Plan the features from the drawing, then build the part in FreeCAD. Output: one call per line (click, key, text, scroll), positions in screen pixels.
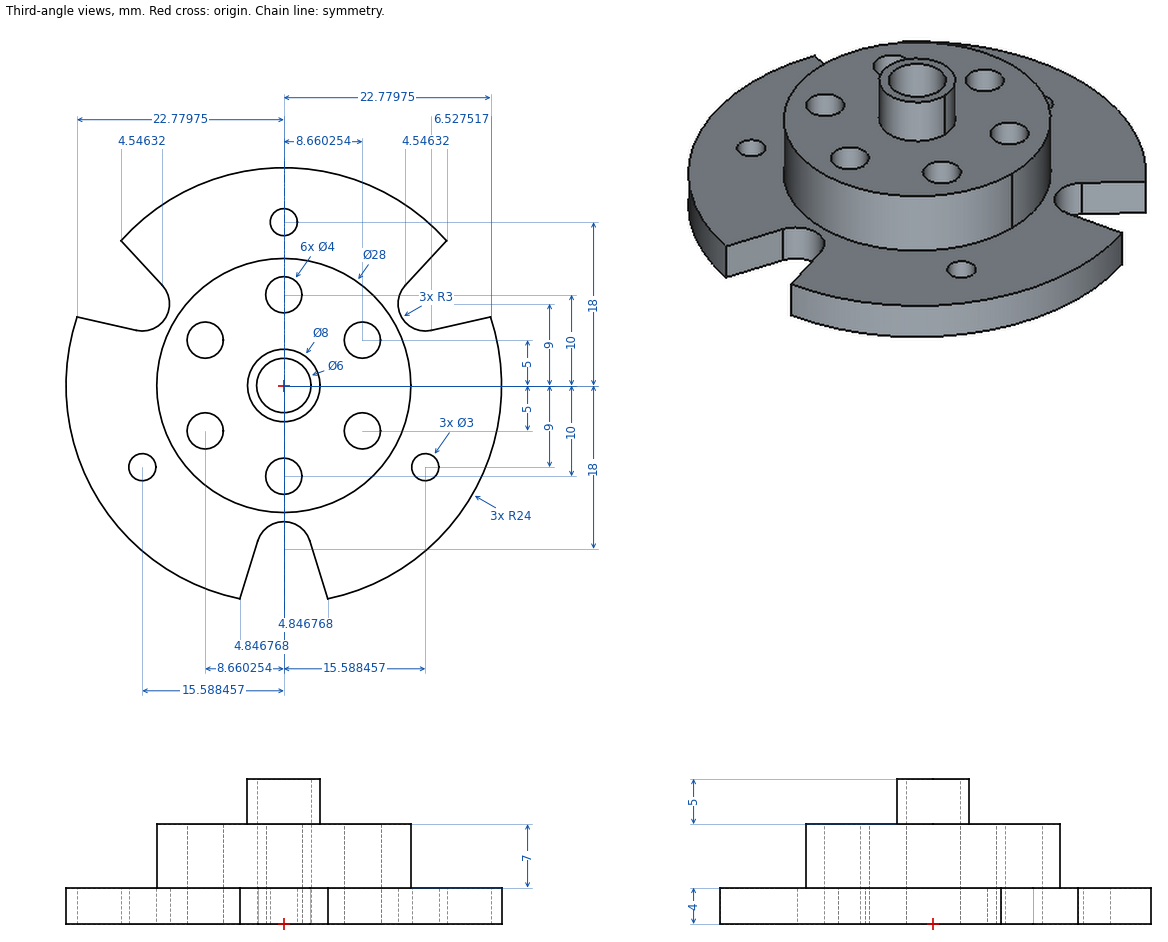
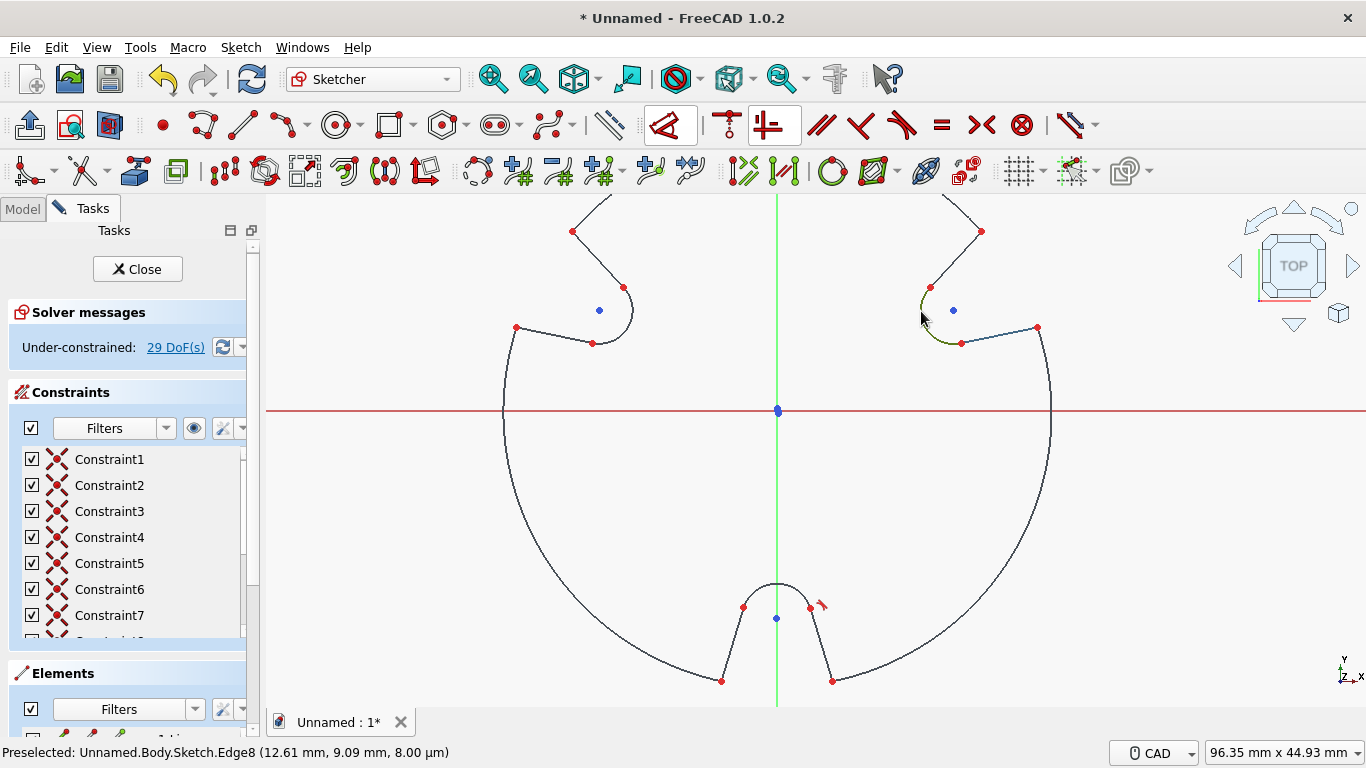
key(t)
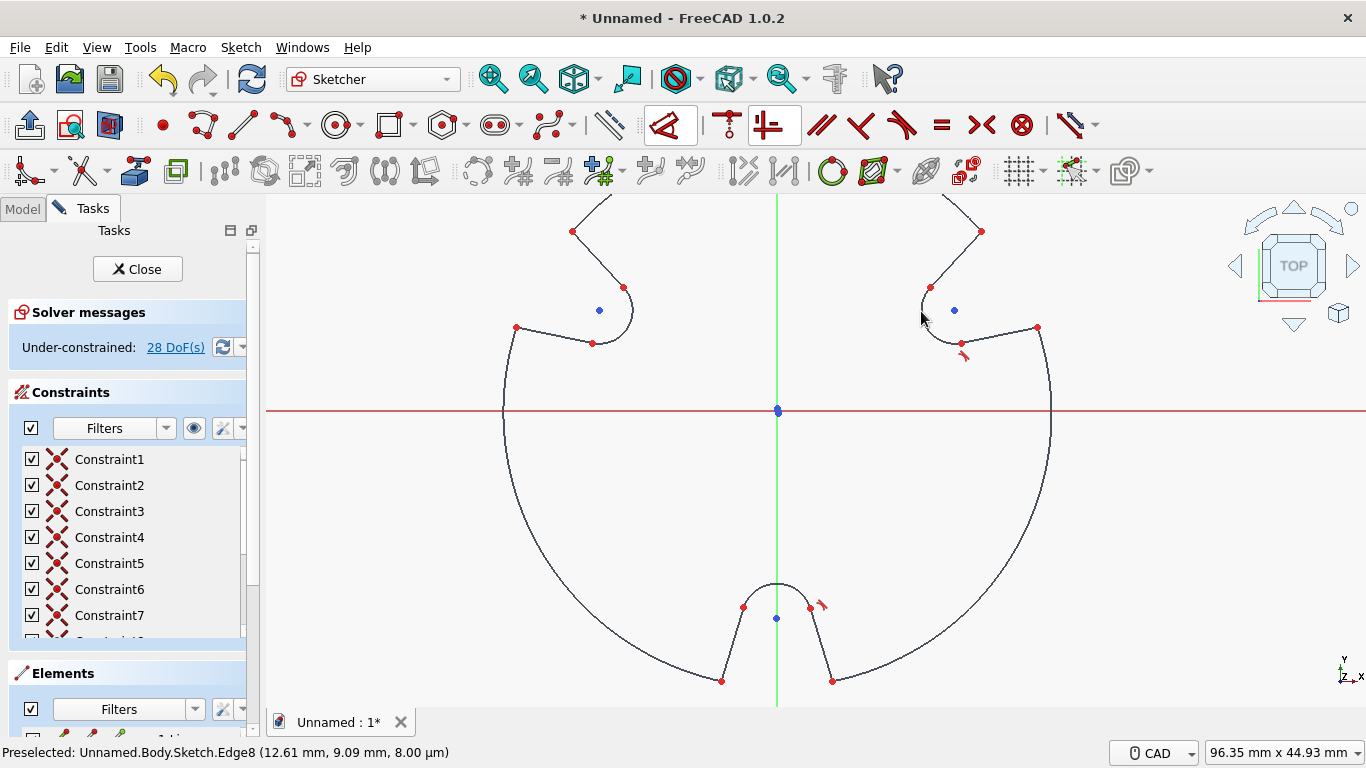
click(946, 271)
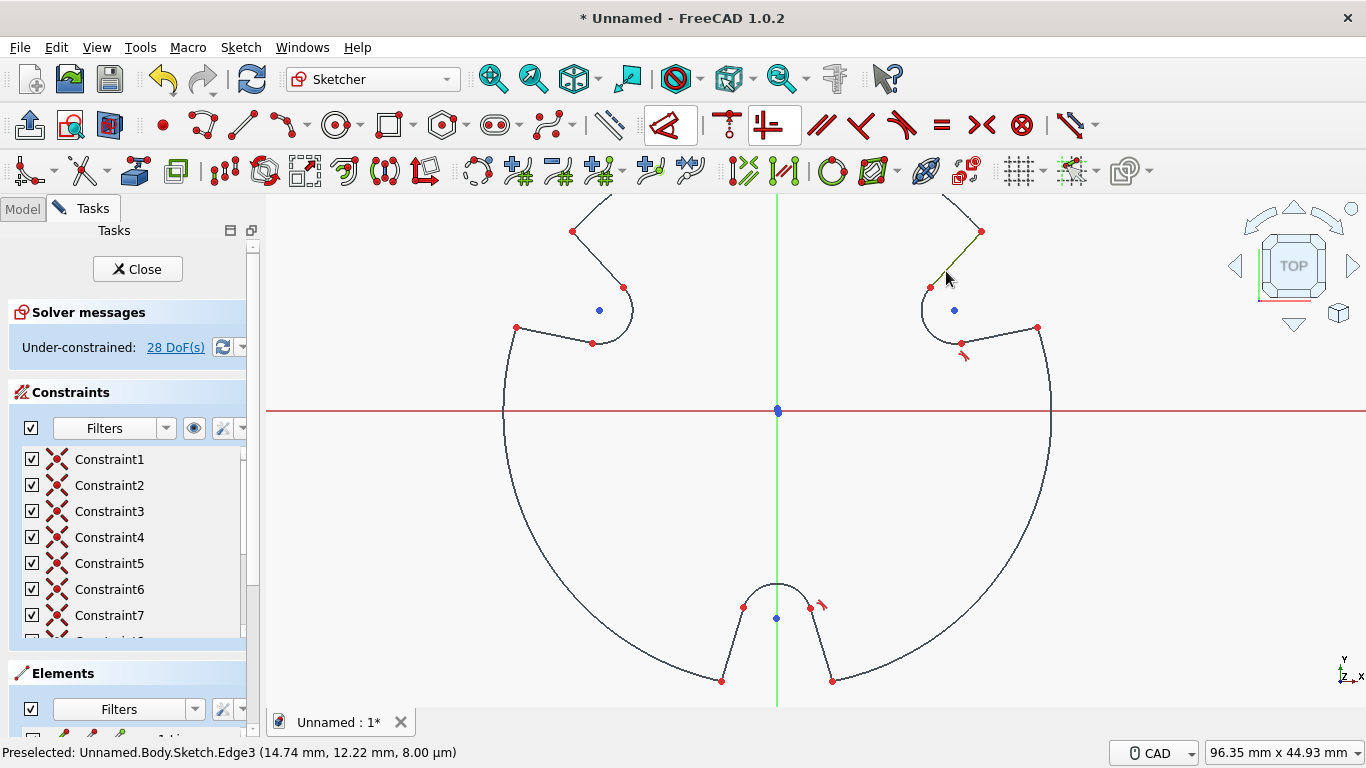
click(922, 310)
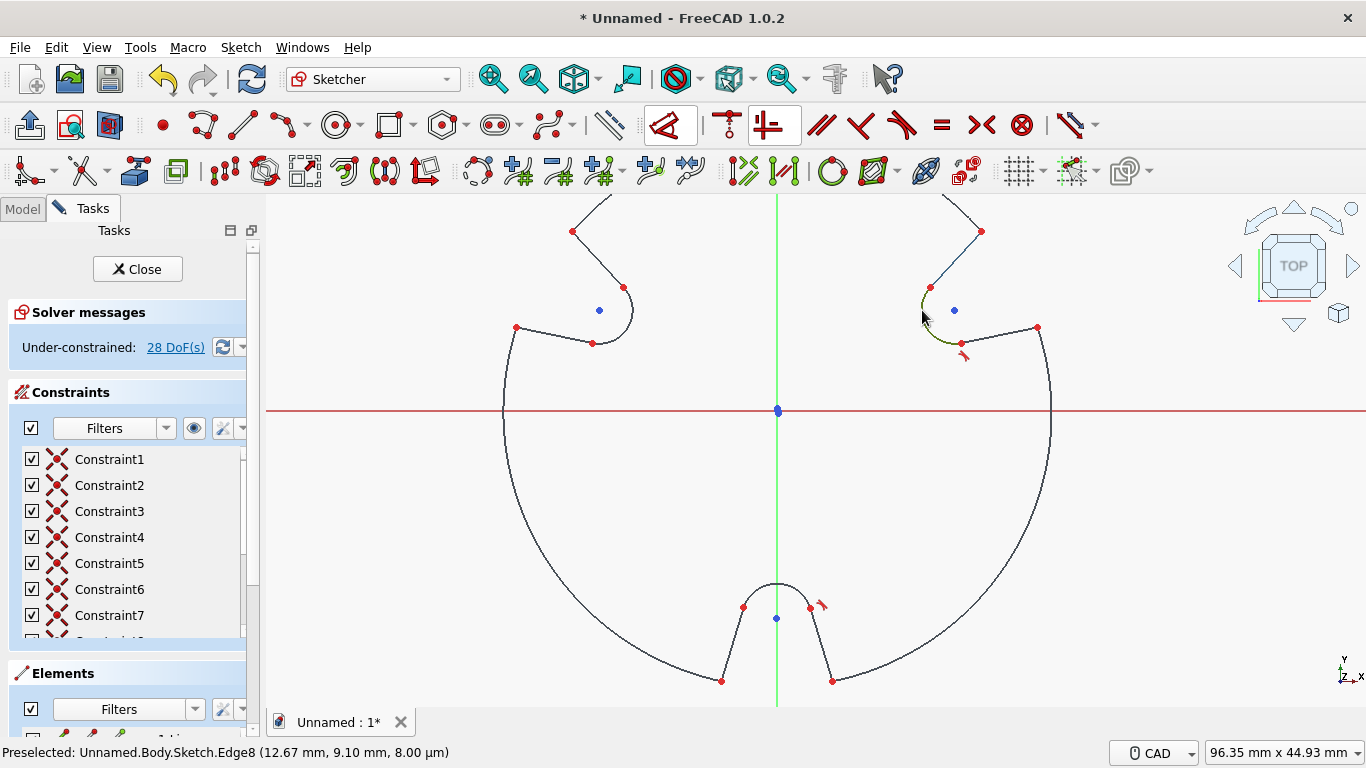
key(t)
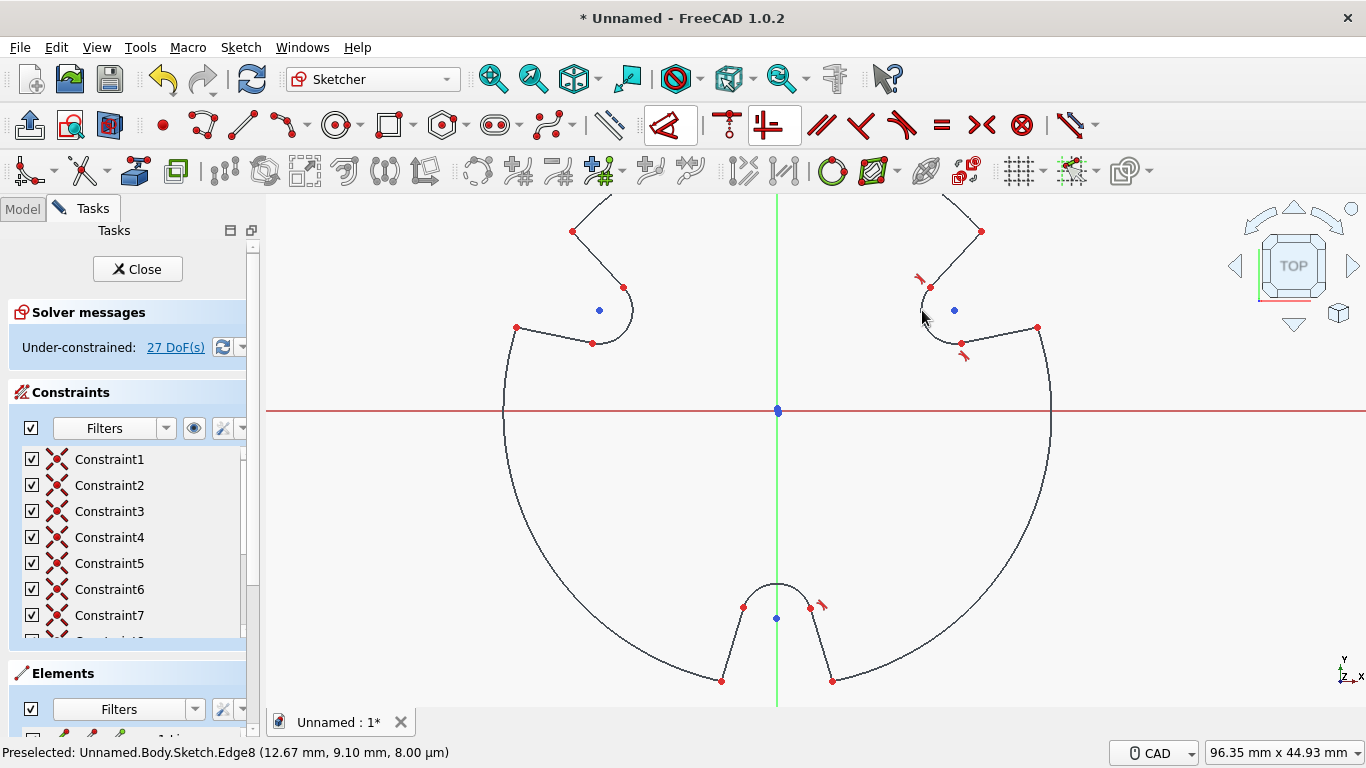
click(588, 248)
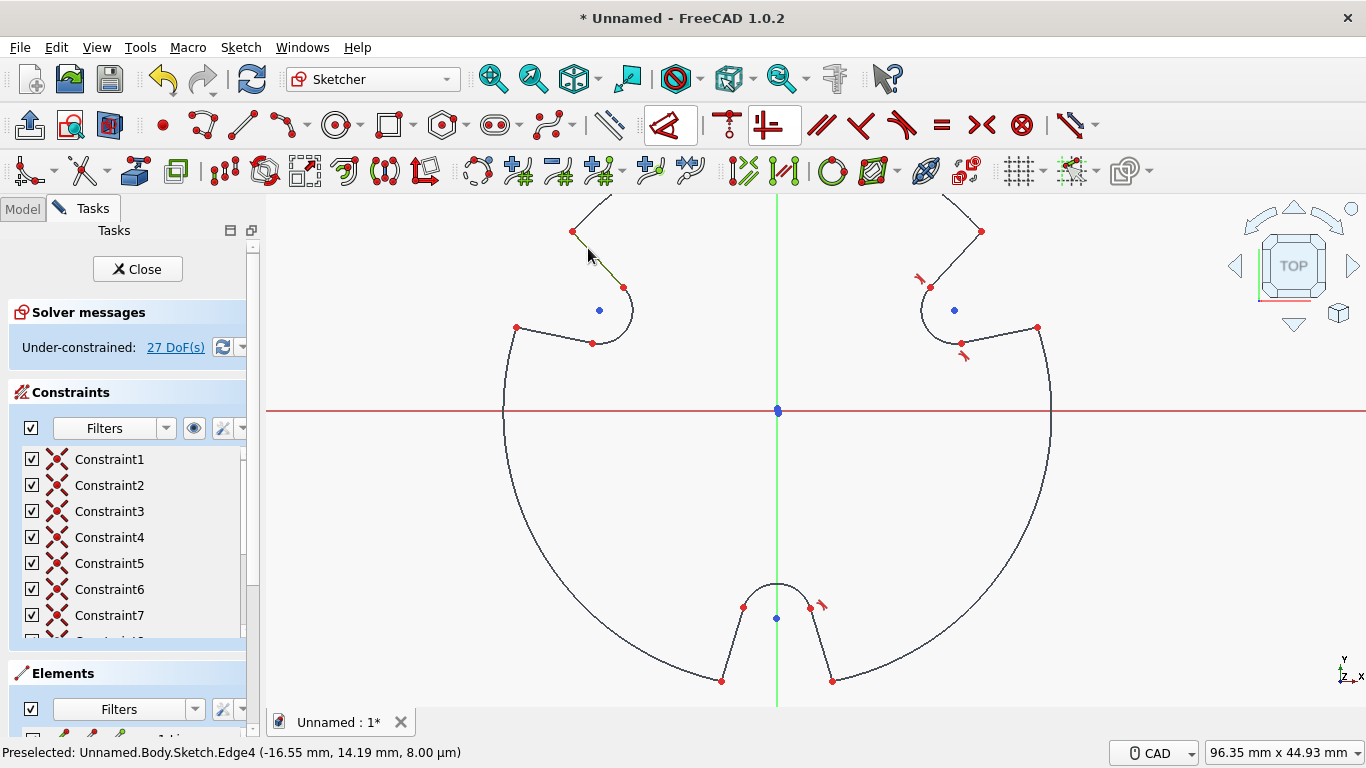
click(617, 339)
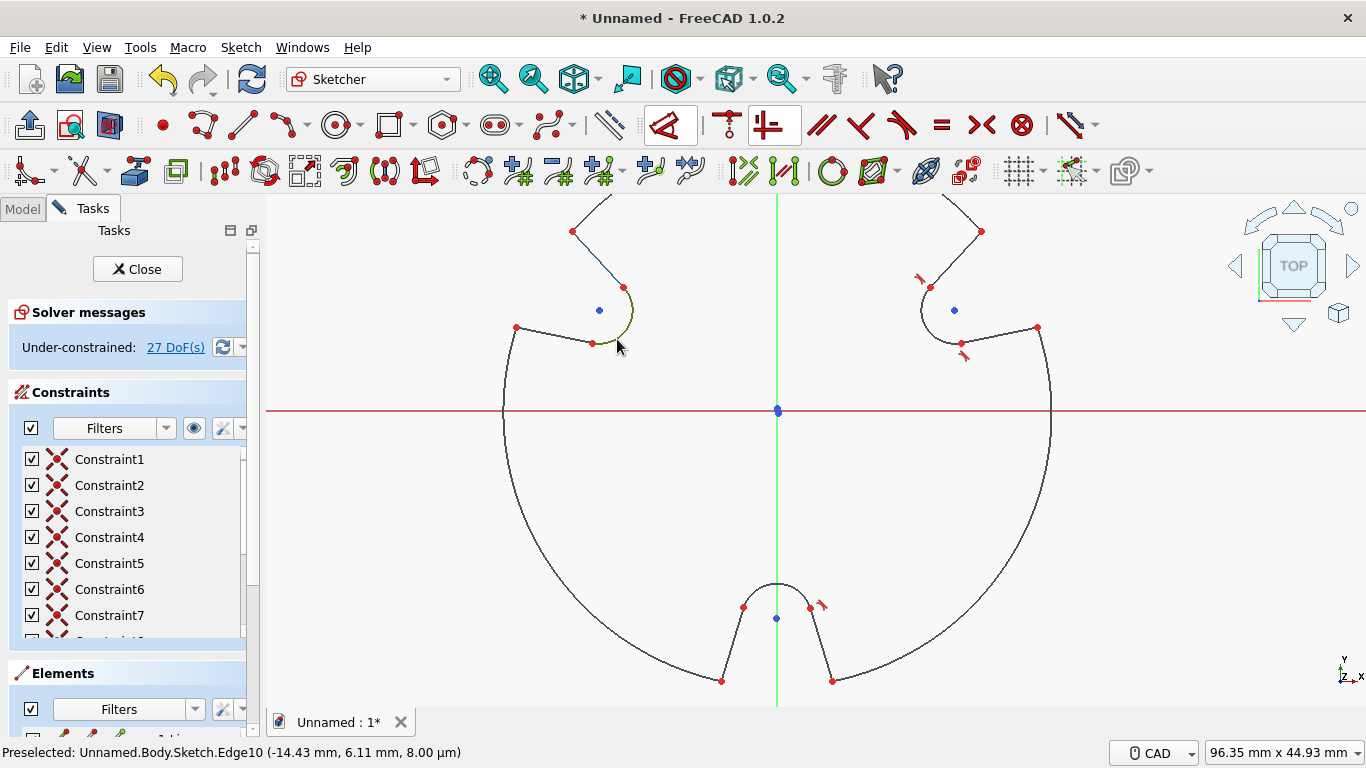
click(902, 126)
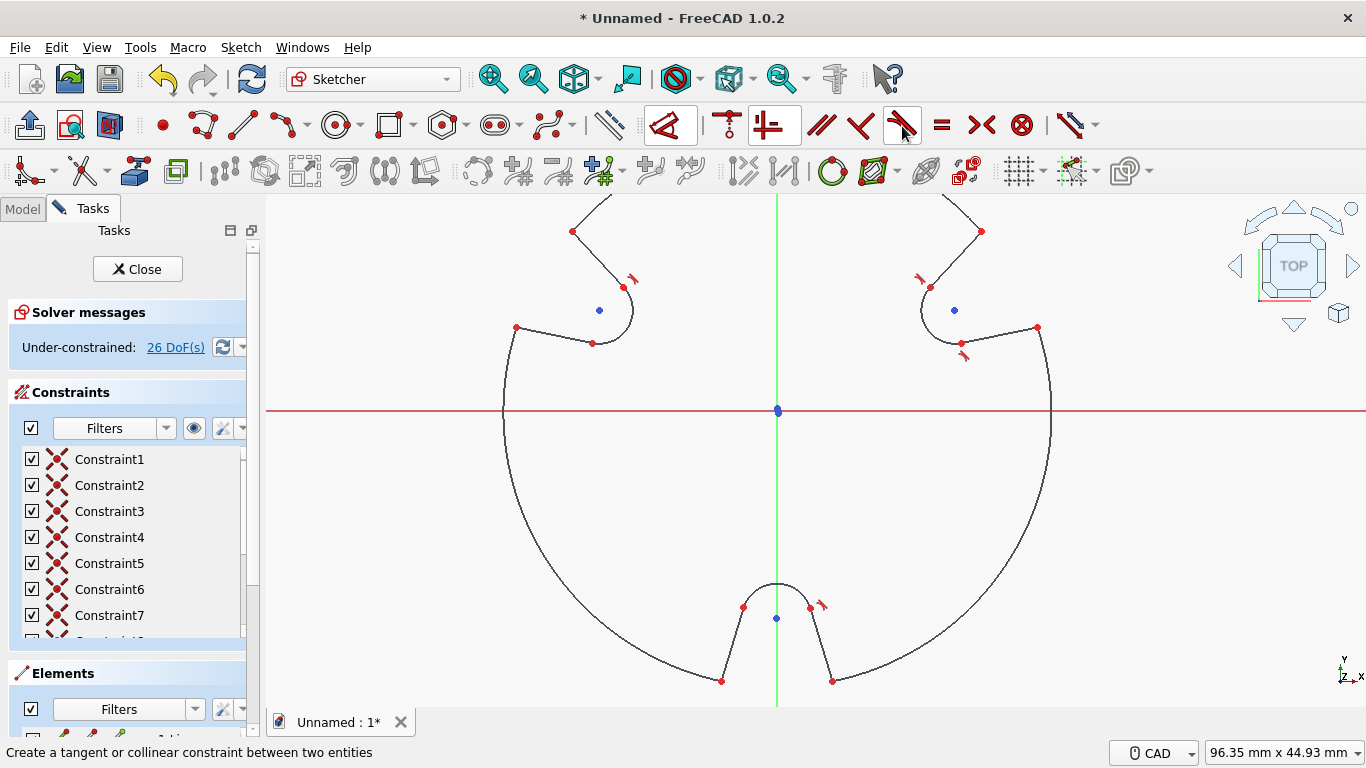
click(570, 338)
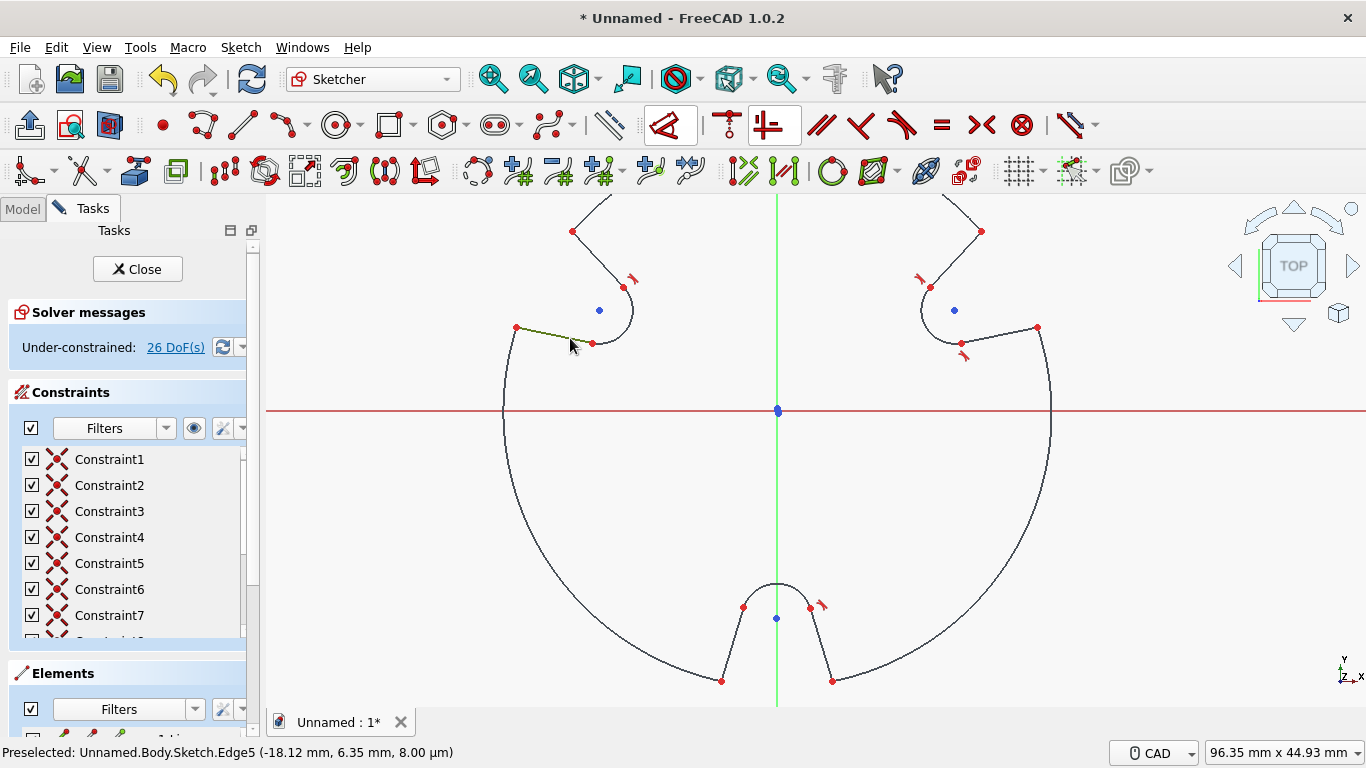
click(617, 339)